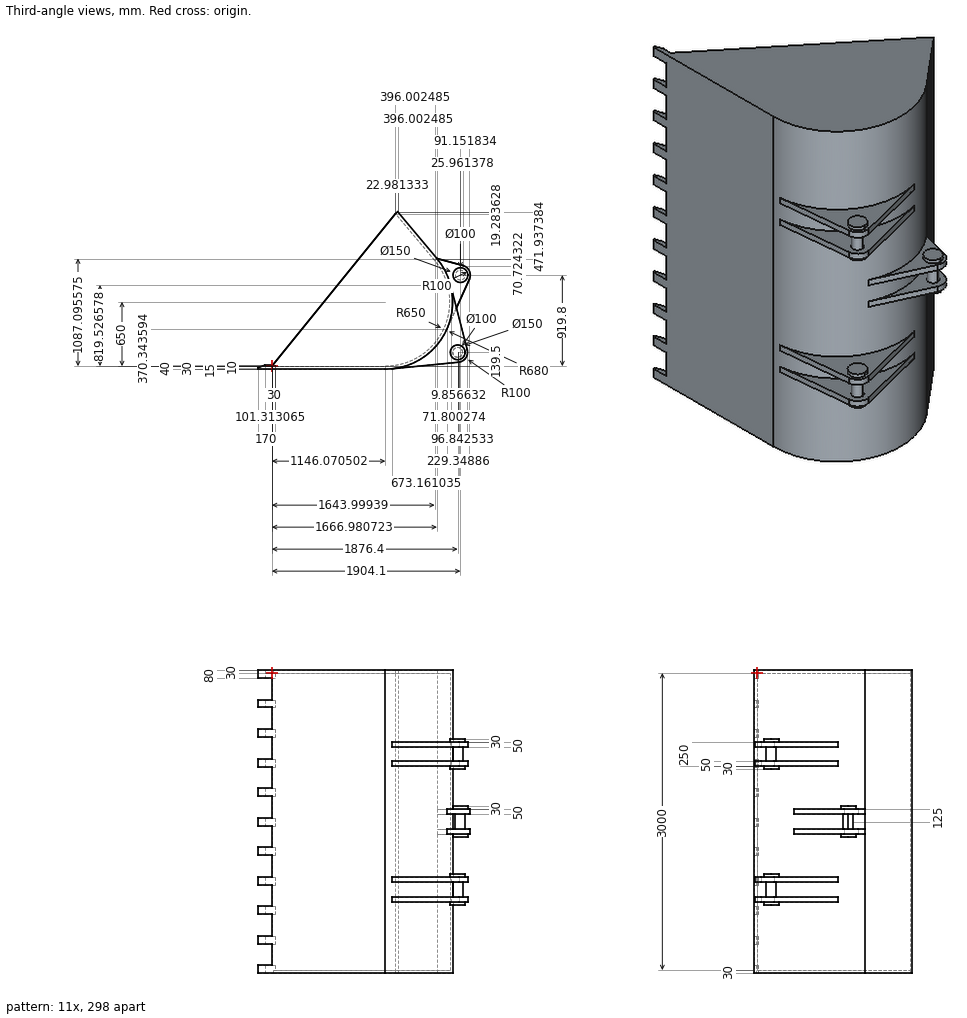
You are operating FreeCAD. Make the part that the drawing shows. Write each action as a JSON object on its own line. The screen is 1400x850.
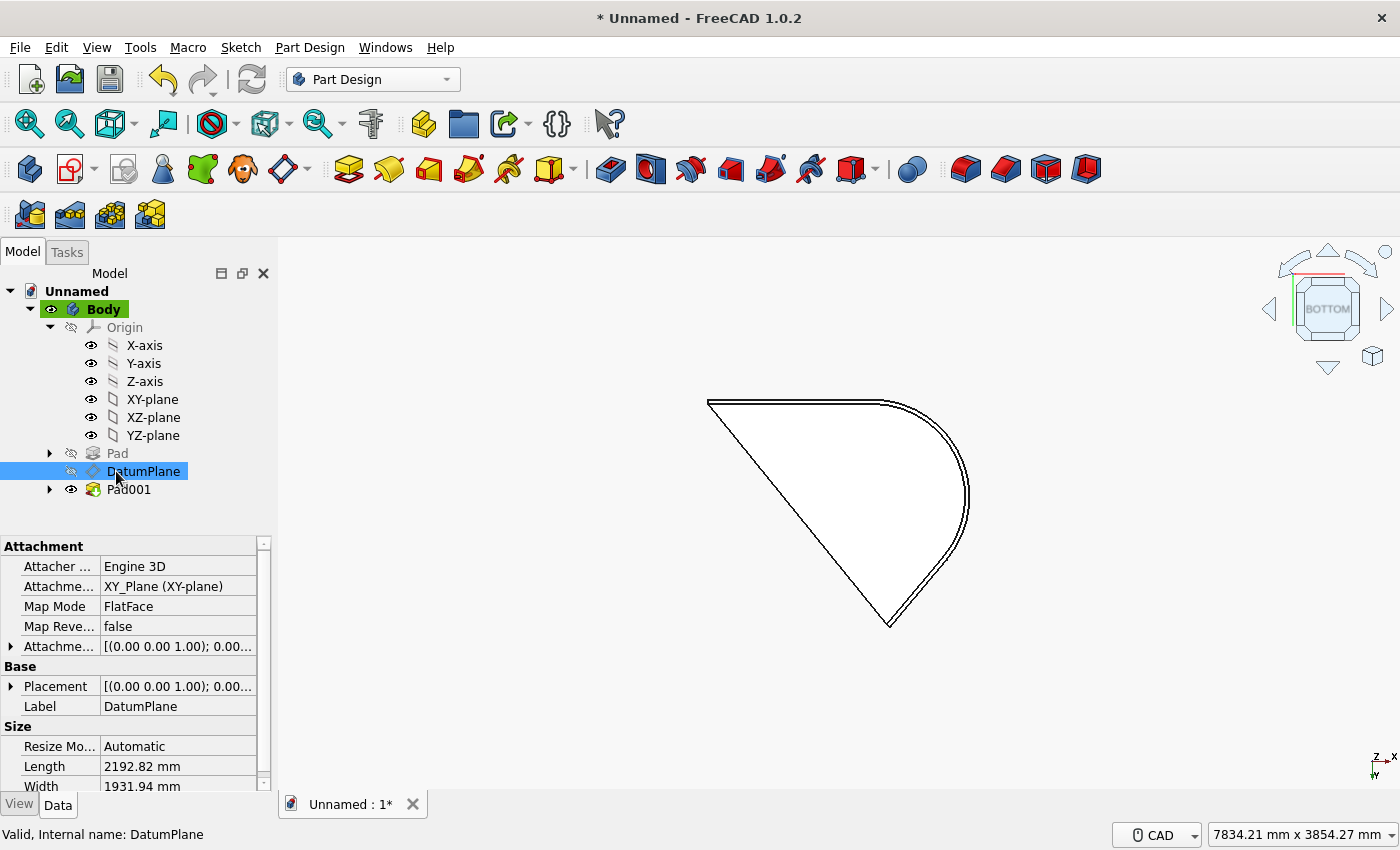
{"action": "key", "text": "v f"}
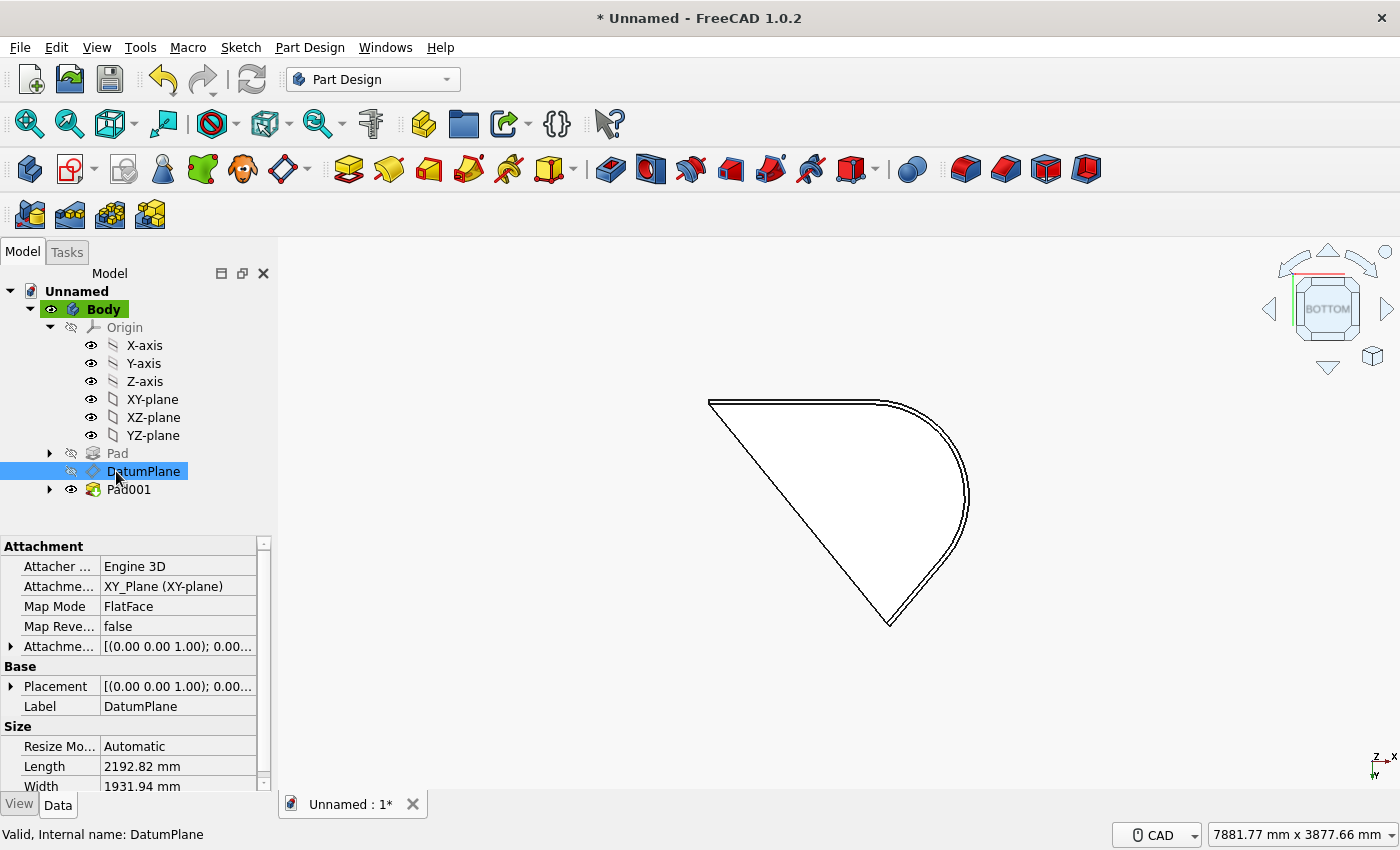
{"action": "scroll", "coordinate": [968, 500], "scroll_direction": "up", "scroll_amount": 11}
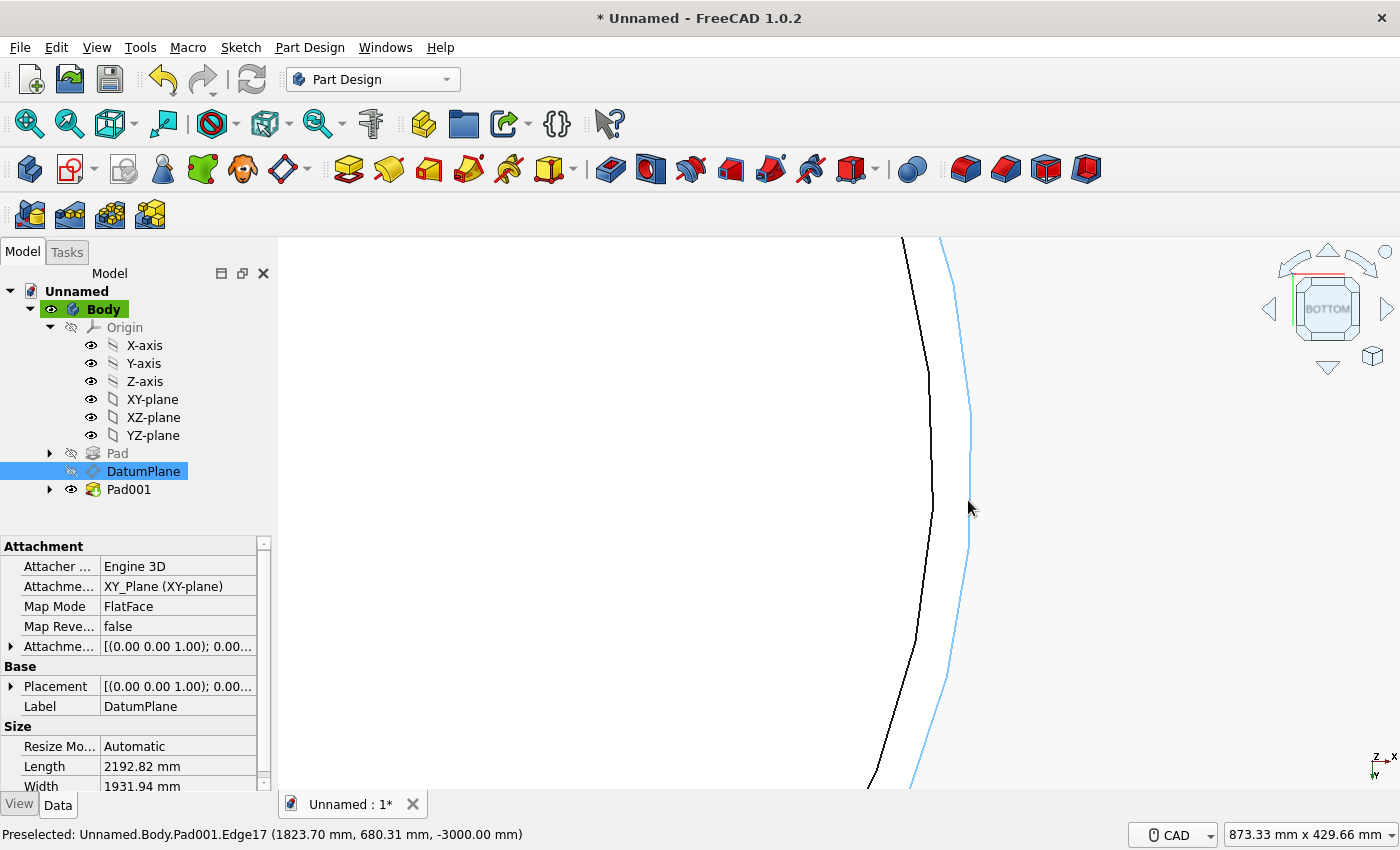
{"action": "left_click", "coordinate": [959, 500]}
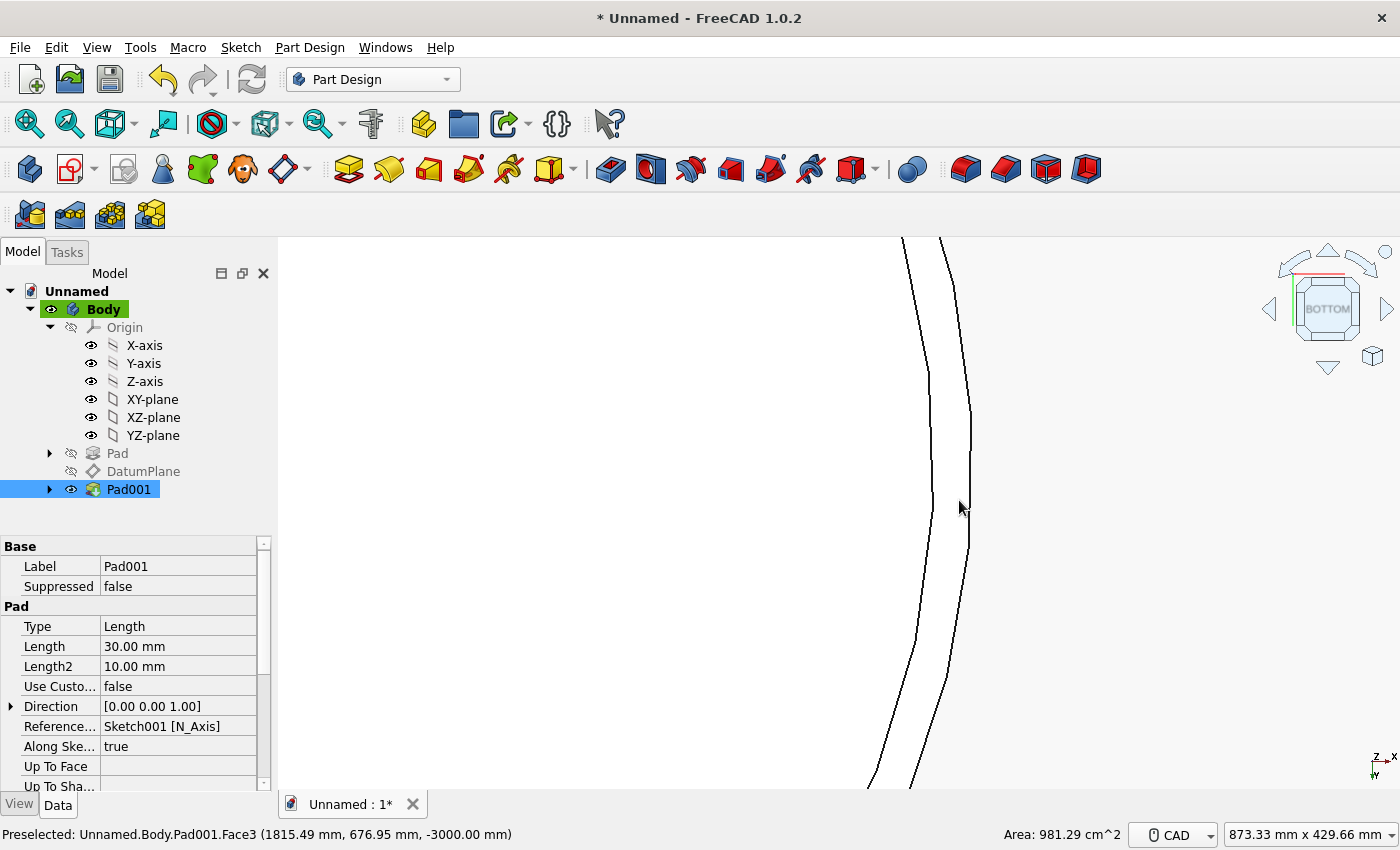
{"action": "left_click", "coordinate": [70, 170]}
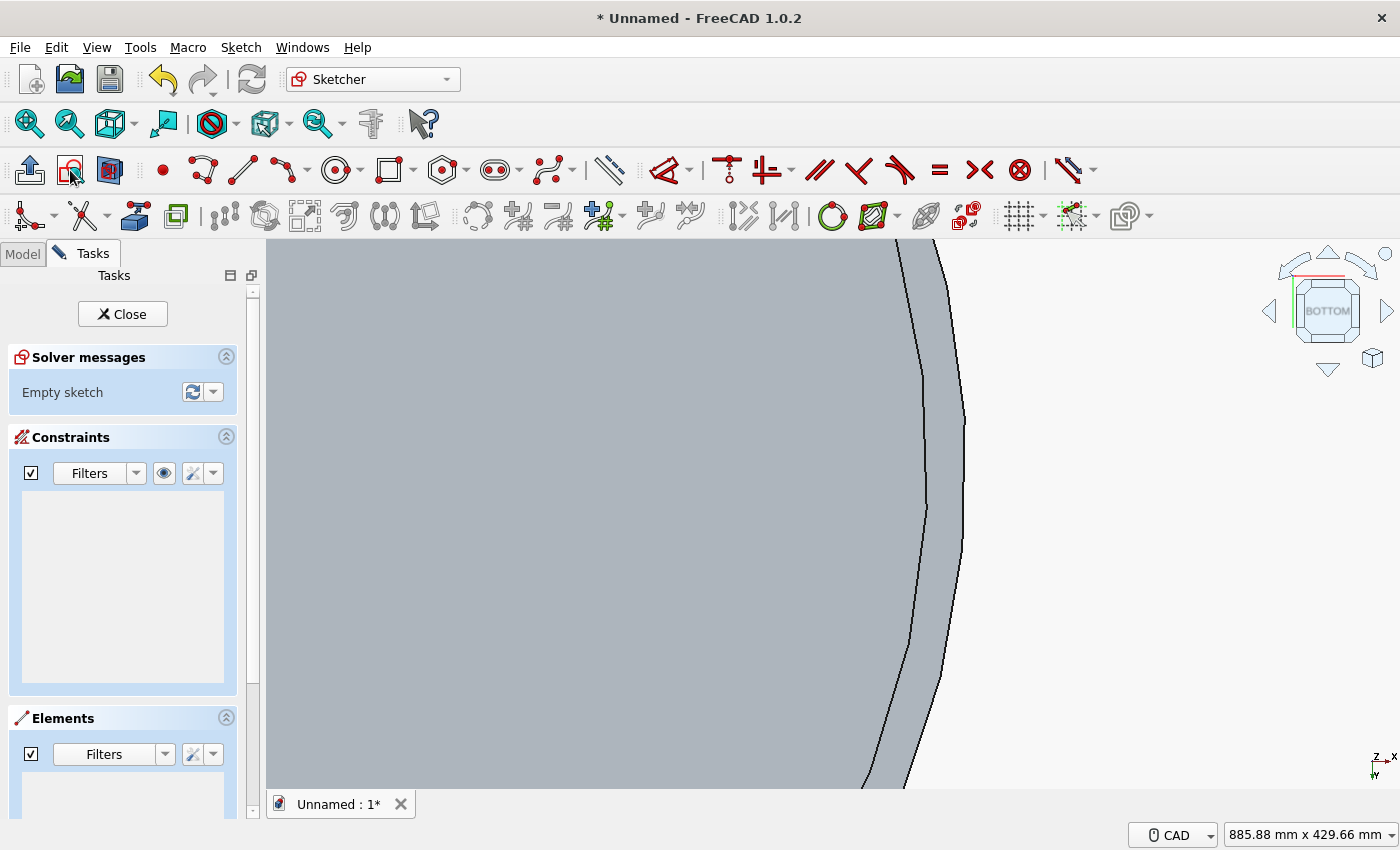
{"action": "scroll", "coordinate": [964, 494], "scroll_direction": "down", "scroll_amount": 9}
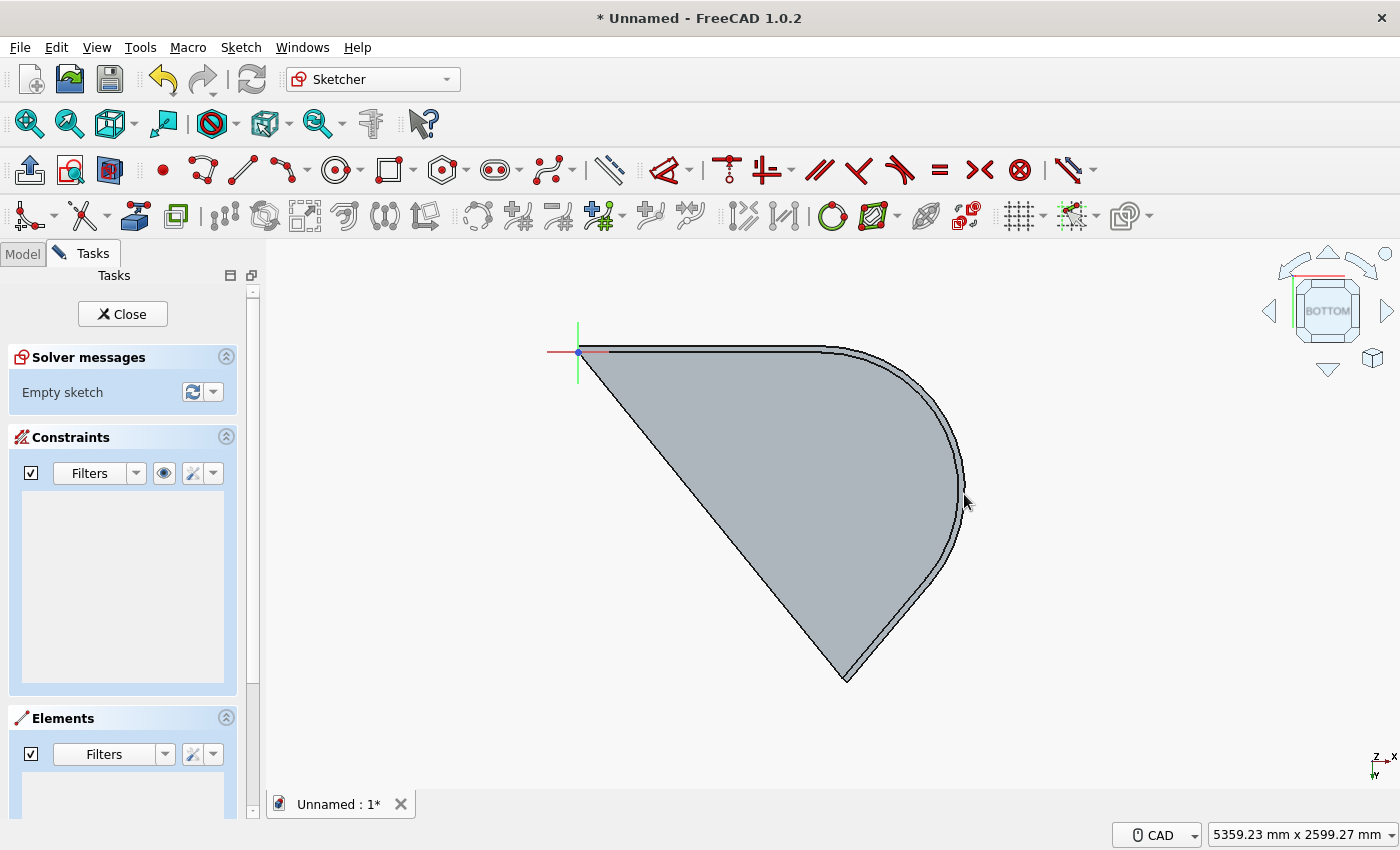
{"action": "left_click", "coordinate": [204, 170]}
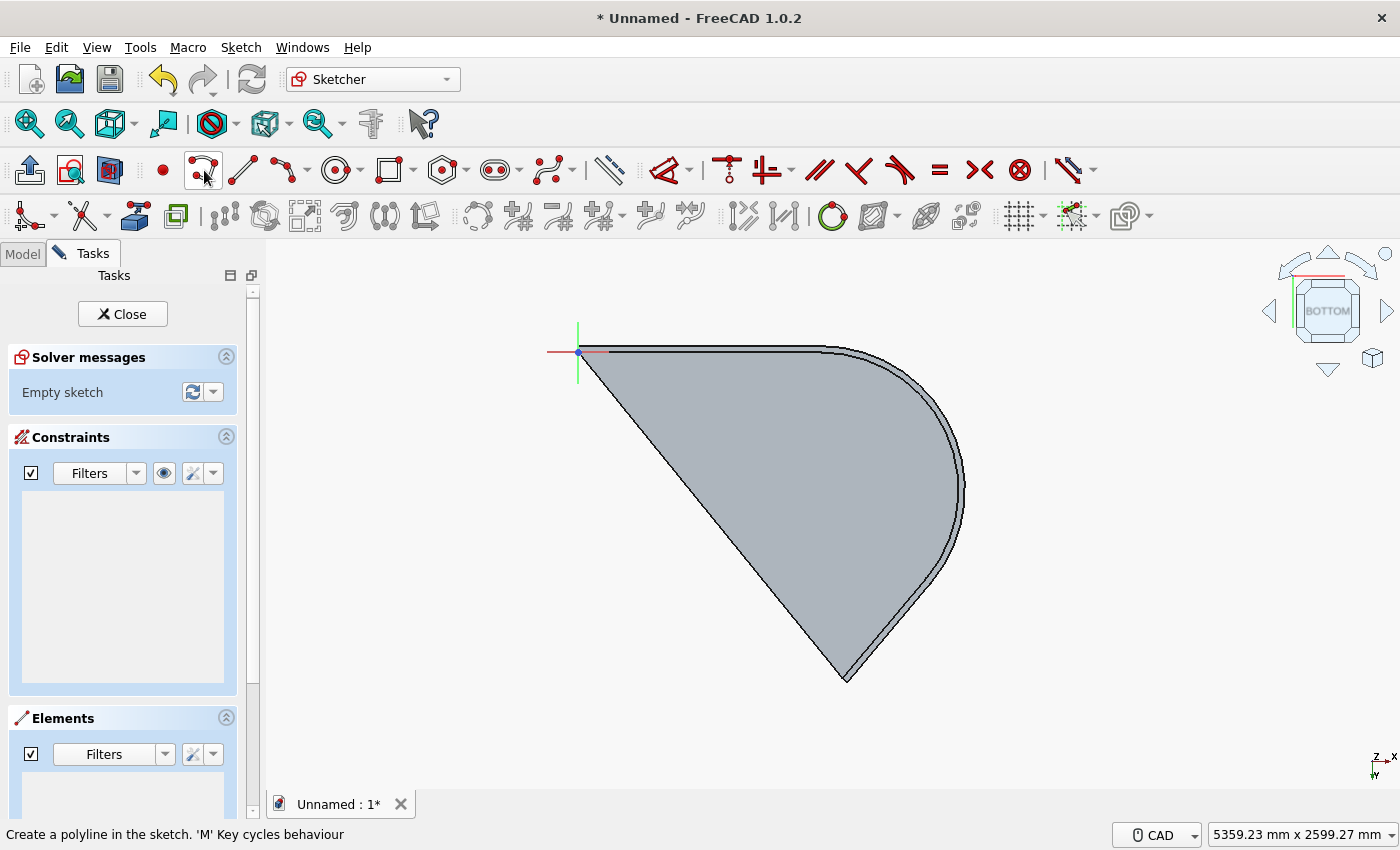
{"action": "left_click", "coordinate": [931, 583]}
{"action": "left_click", "coordinate": [847, 682]}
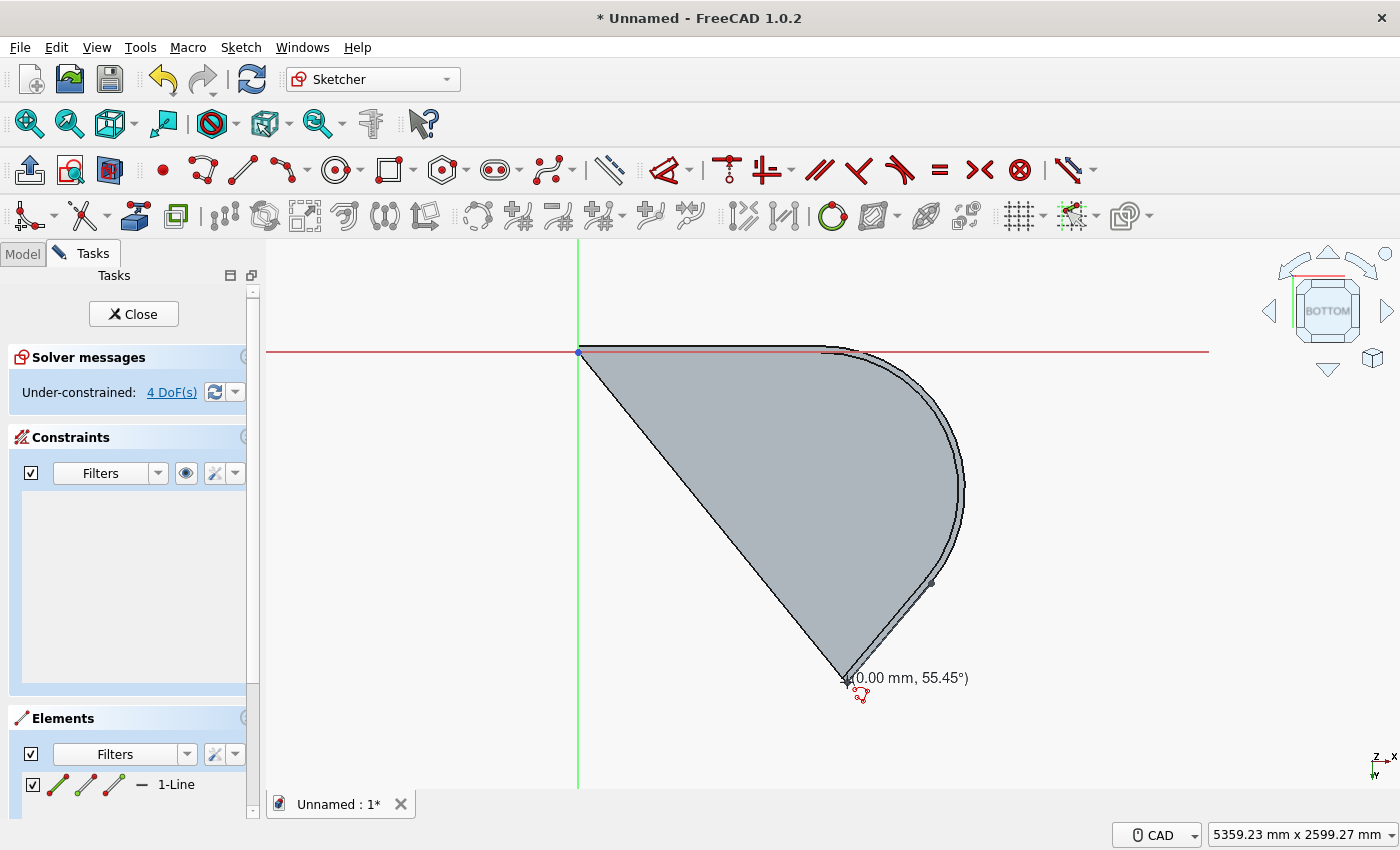
{"action": "scroll", "coordinate": [843, 678], "scroll_direction": "up", "scroll_amount": 5}